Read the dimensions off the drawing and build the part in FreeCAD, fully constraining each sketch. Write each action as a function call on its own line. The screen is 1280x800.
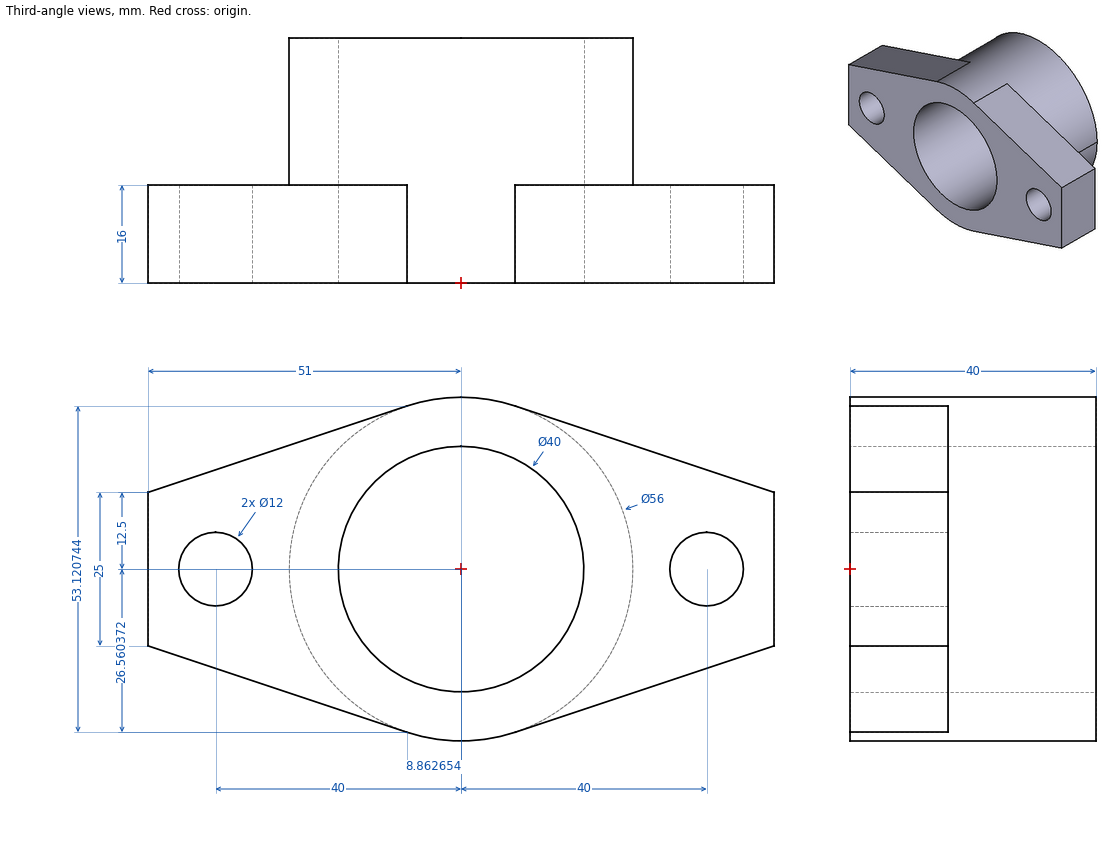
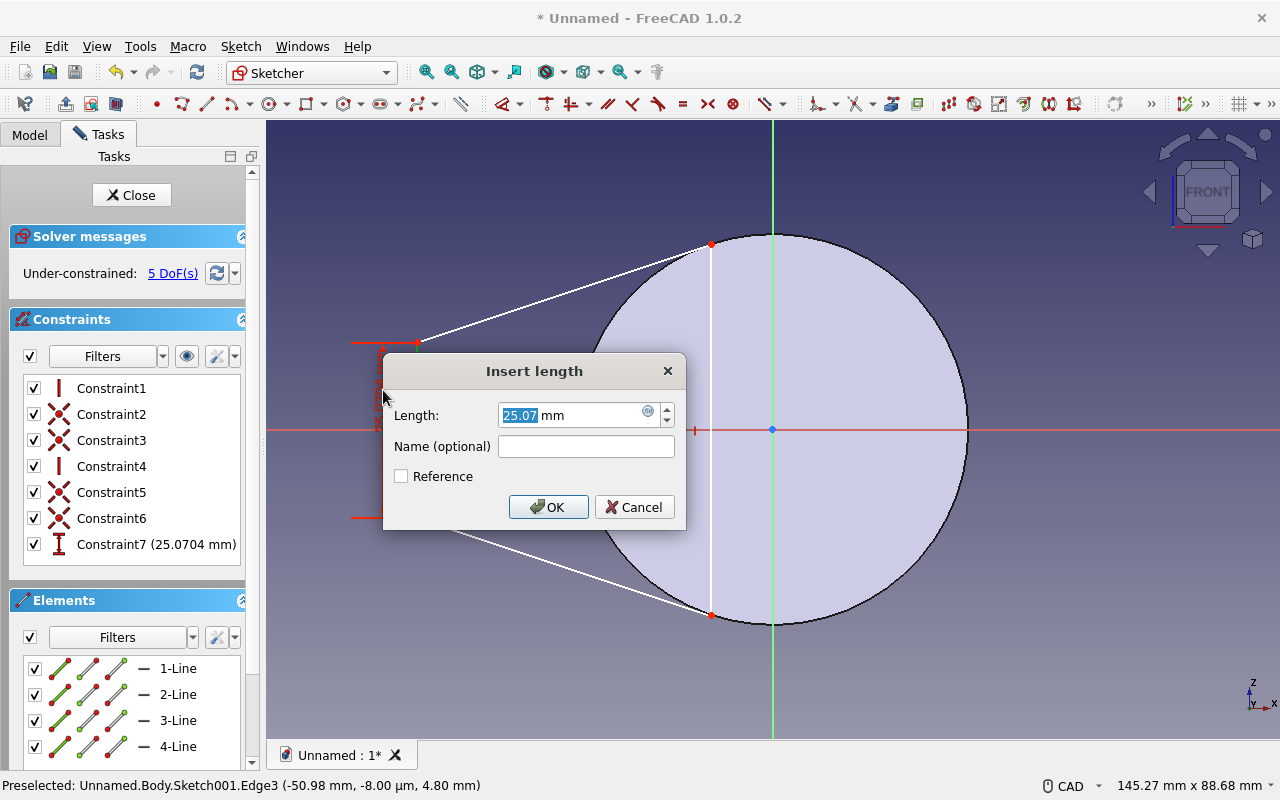
text(25)
key(Return)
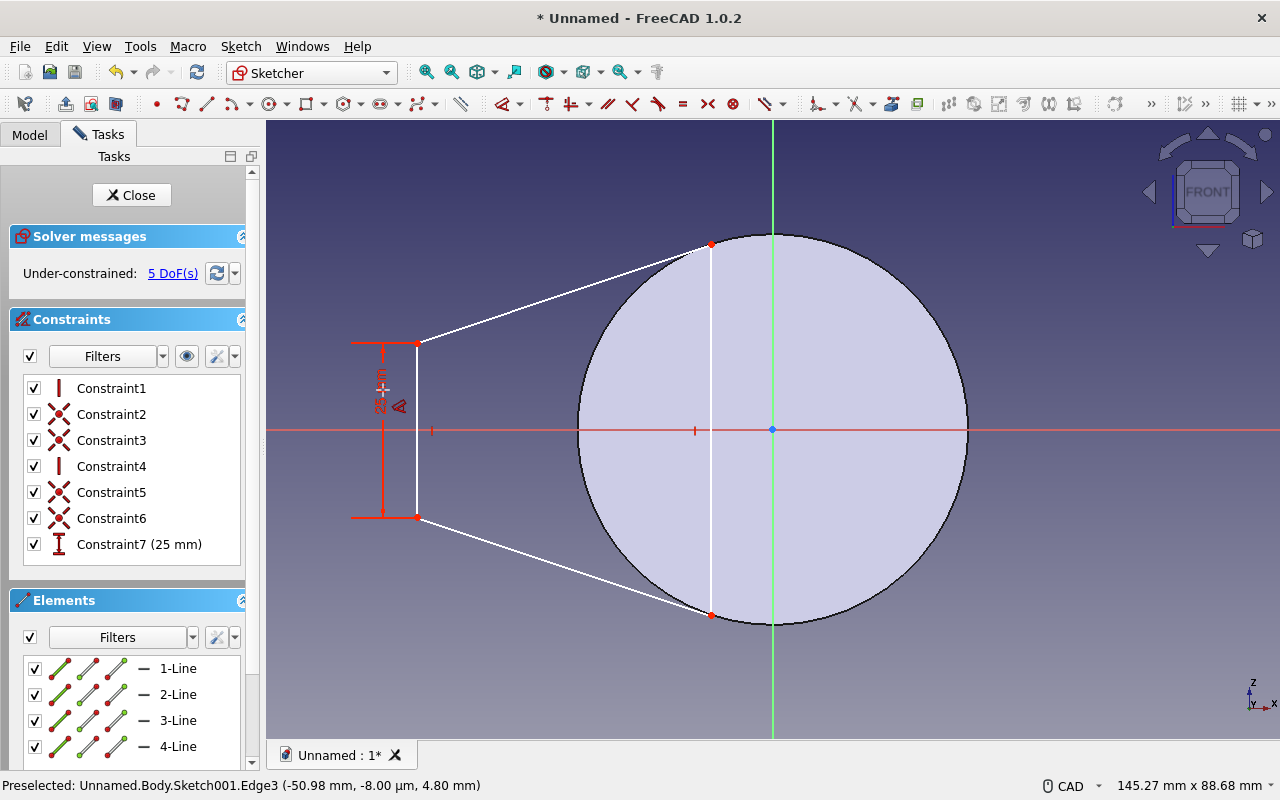
click(417, 343)
click(595, 309)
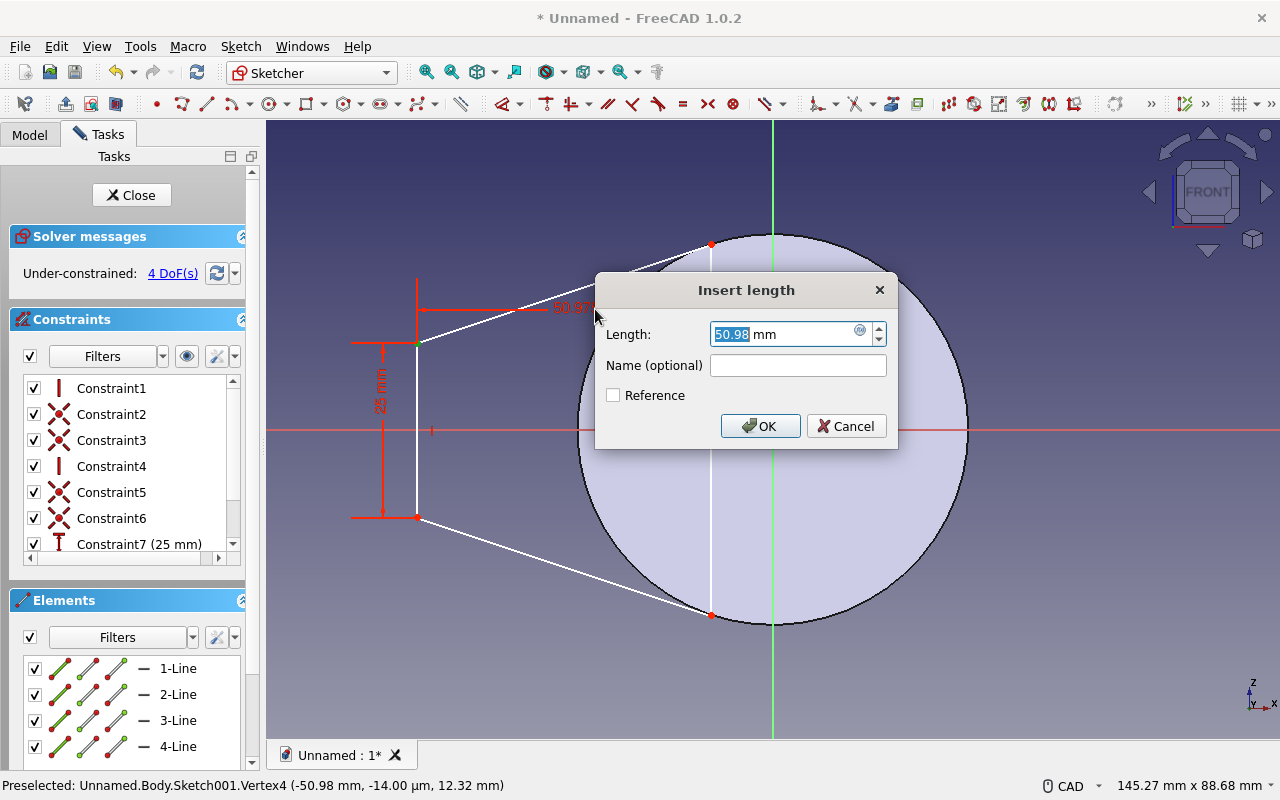
text(51)
key(Return)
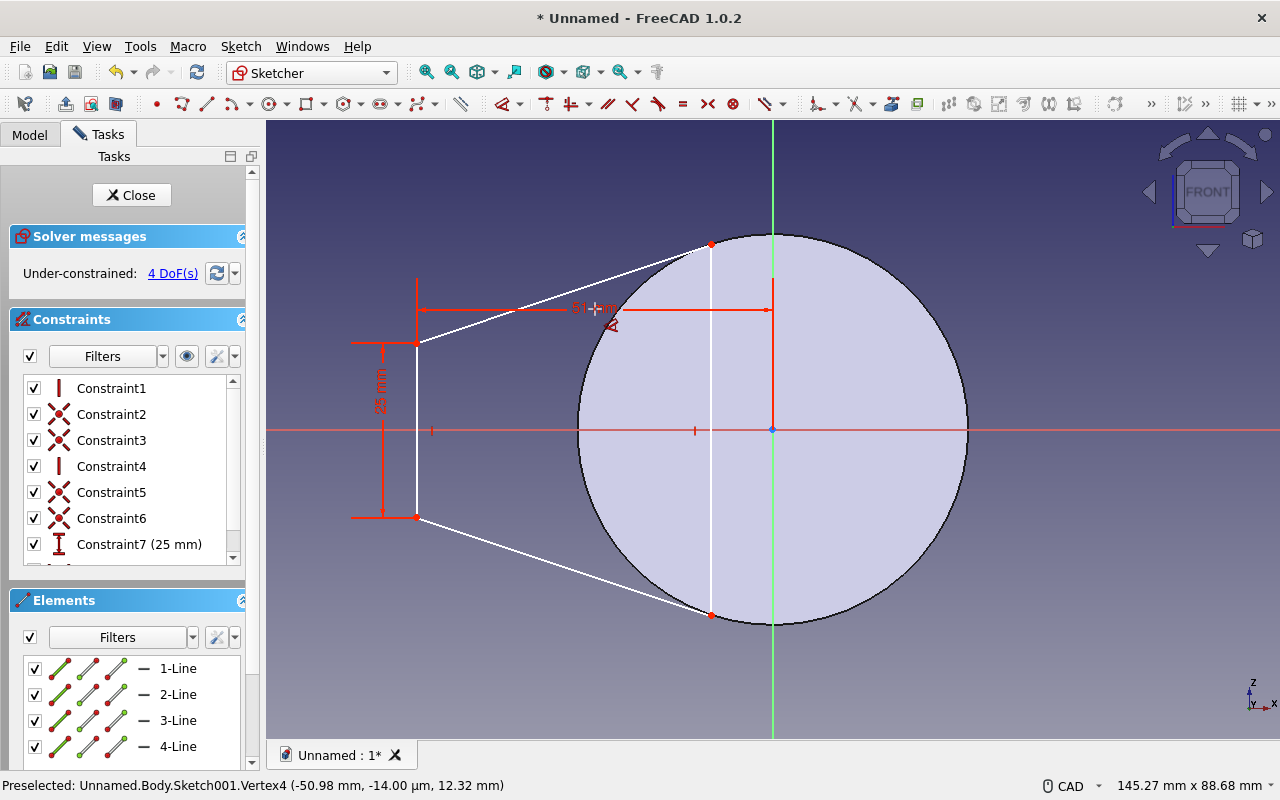
click(417, 343)
click(807, 386)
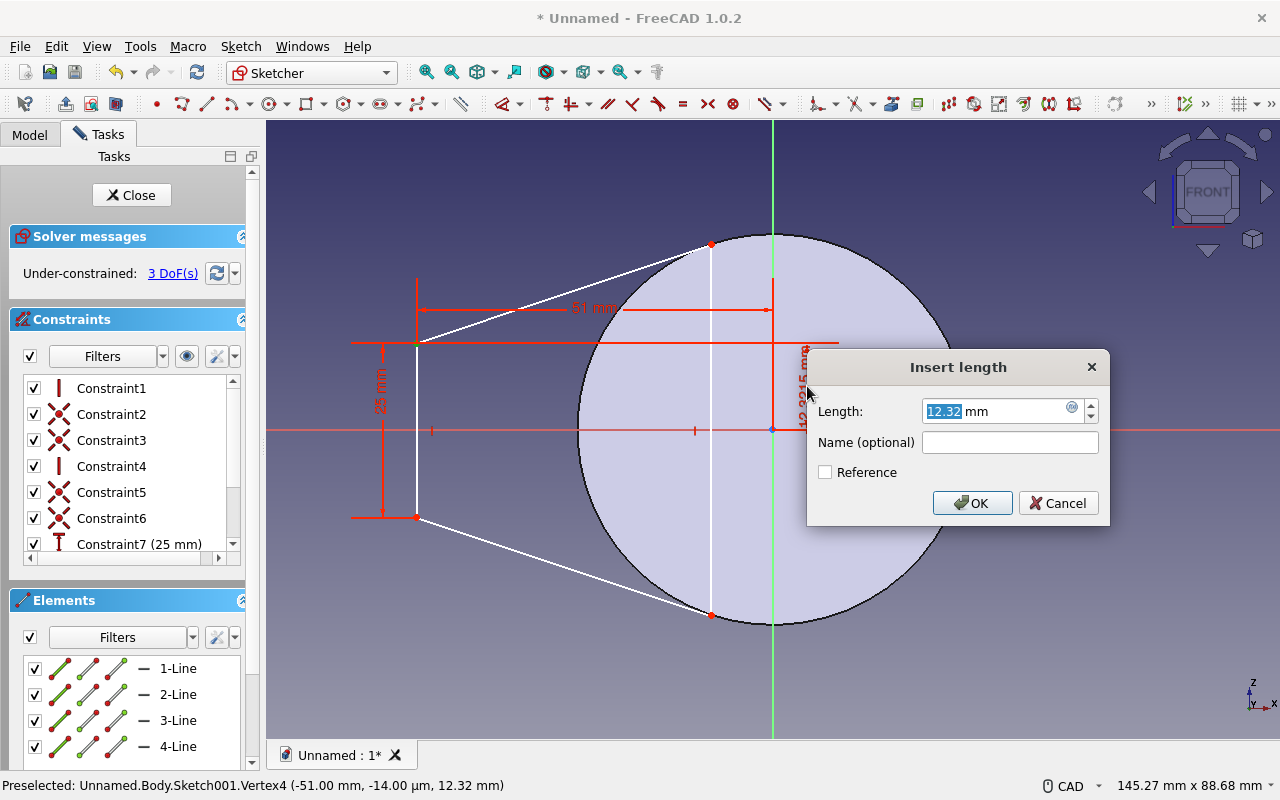
text(12.5)
key(Return)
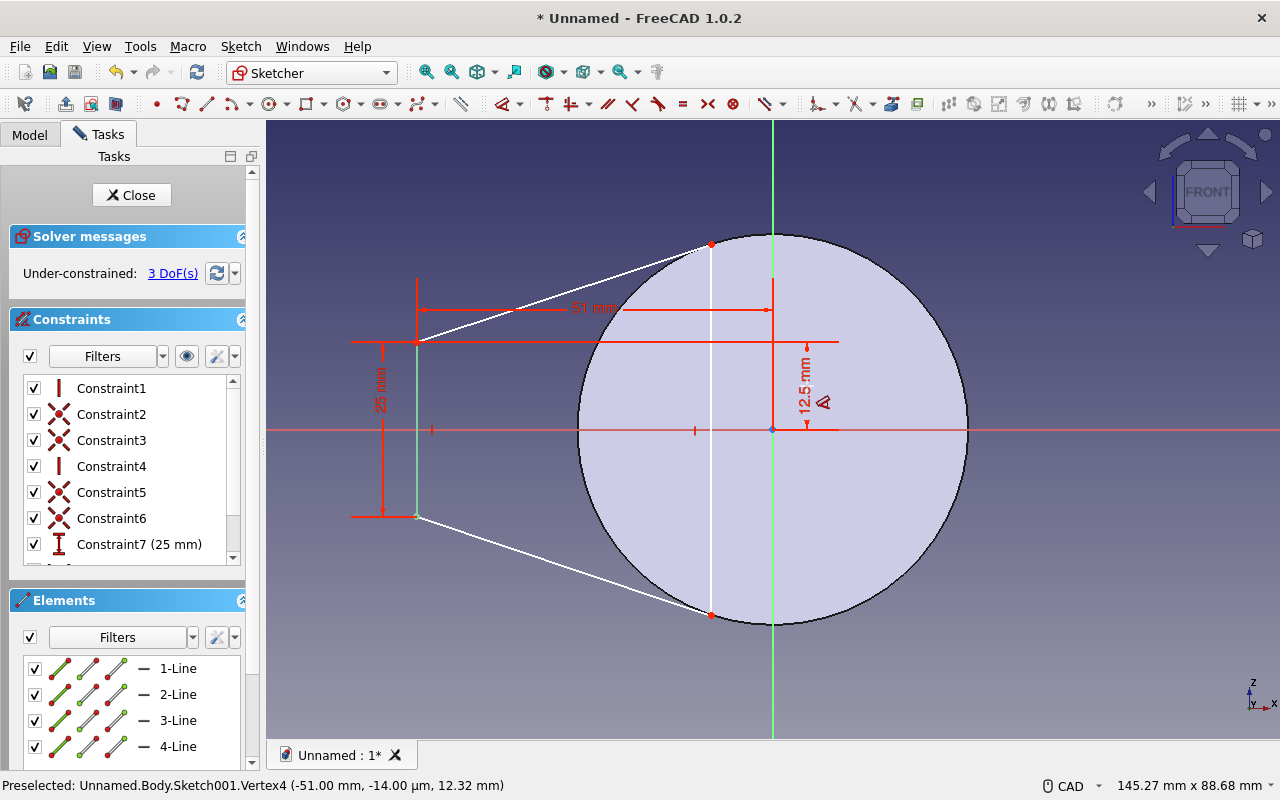
click(711, 505)
click(745, 345)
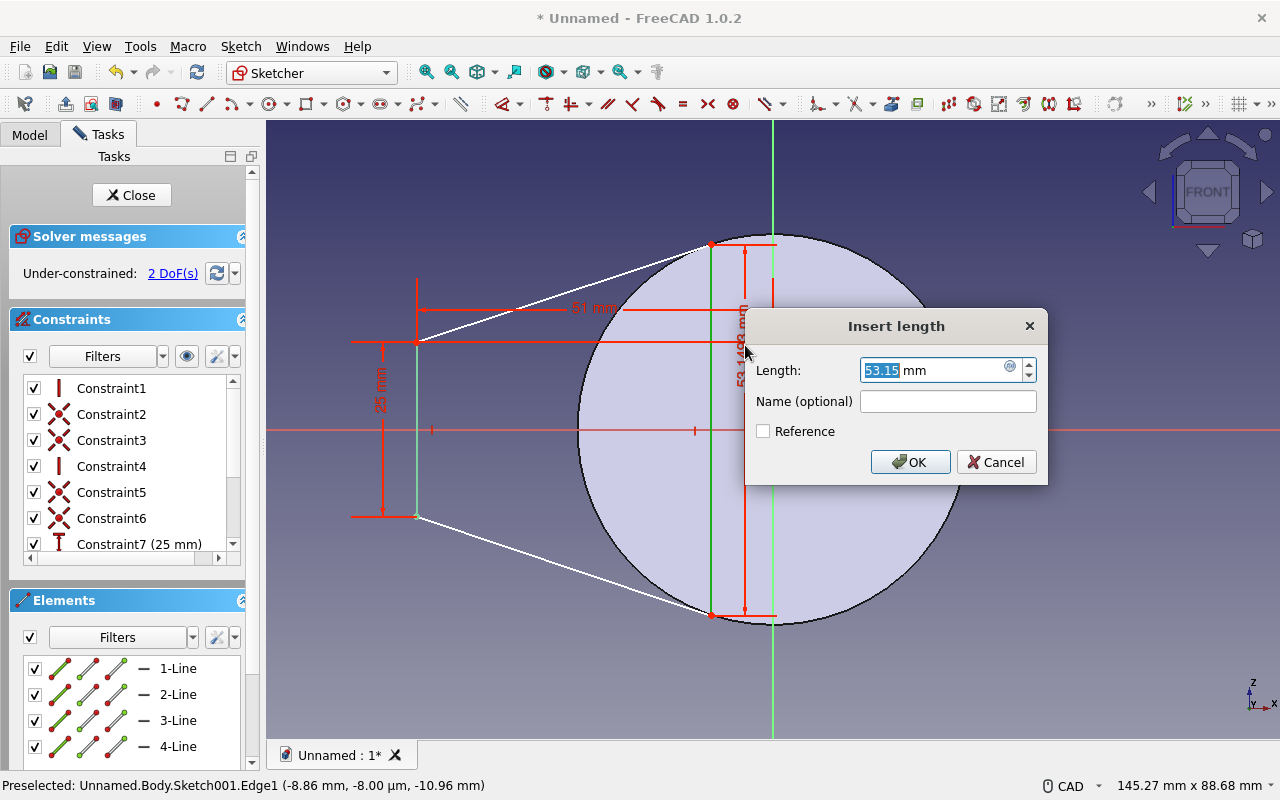
text(53.120744)
key(Return)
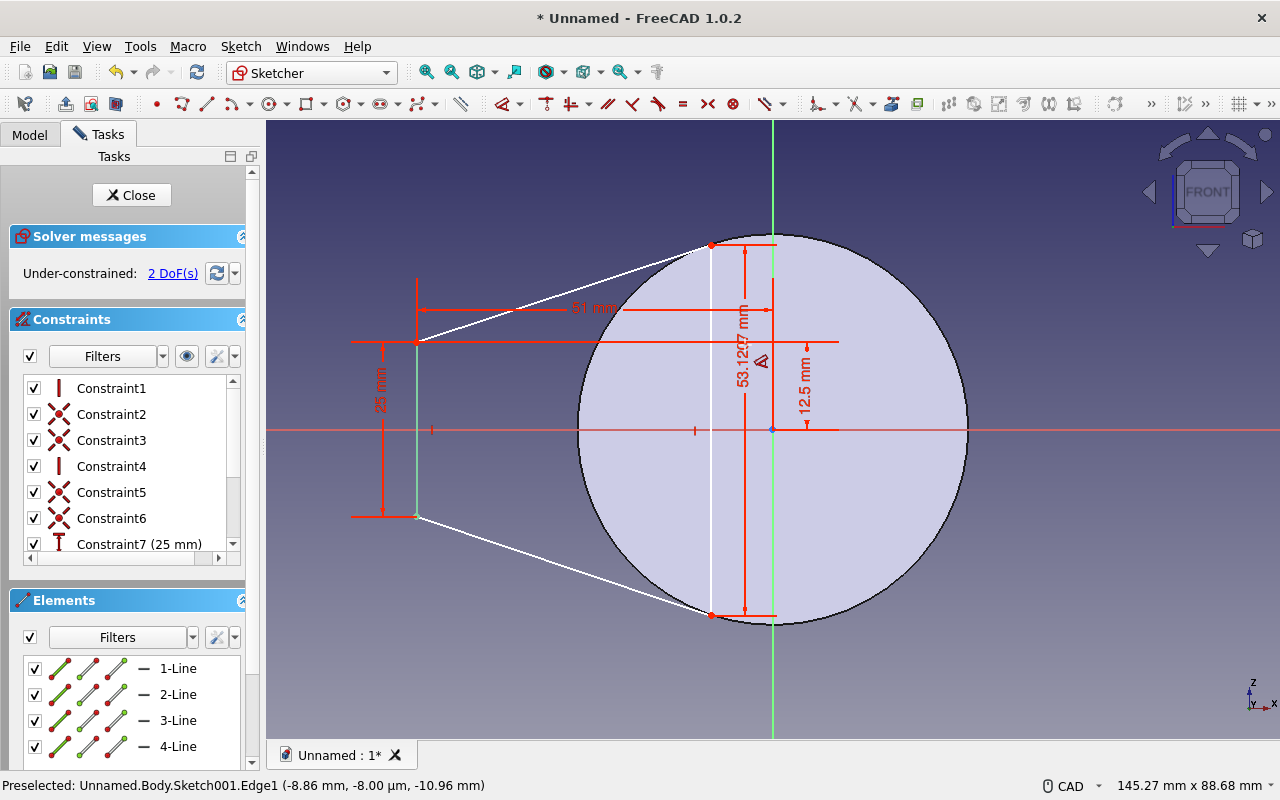
click(711, 616)
click(742, 650)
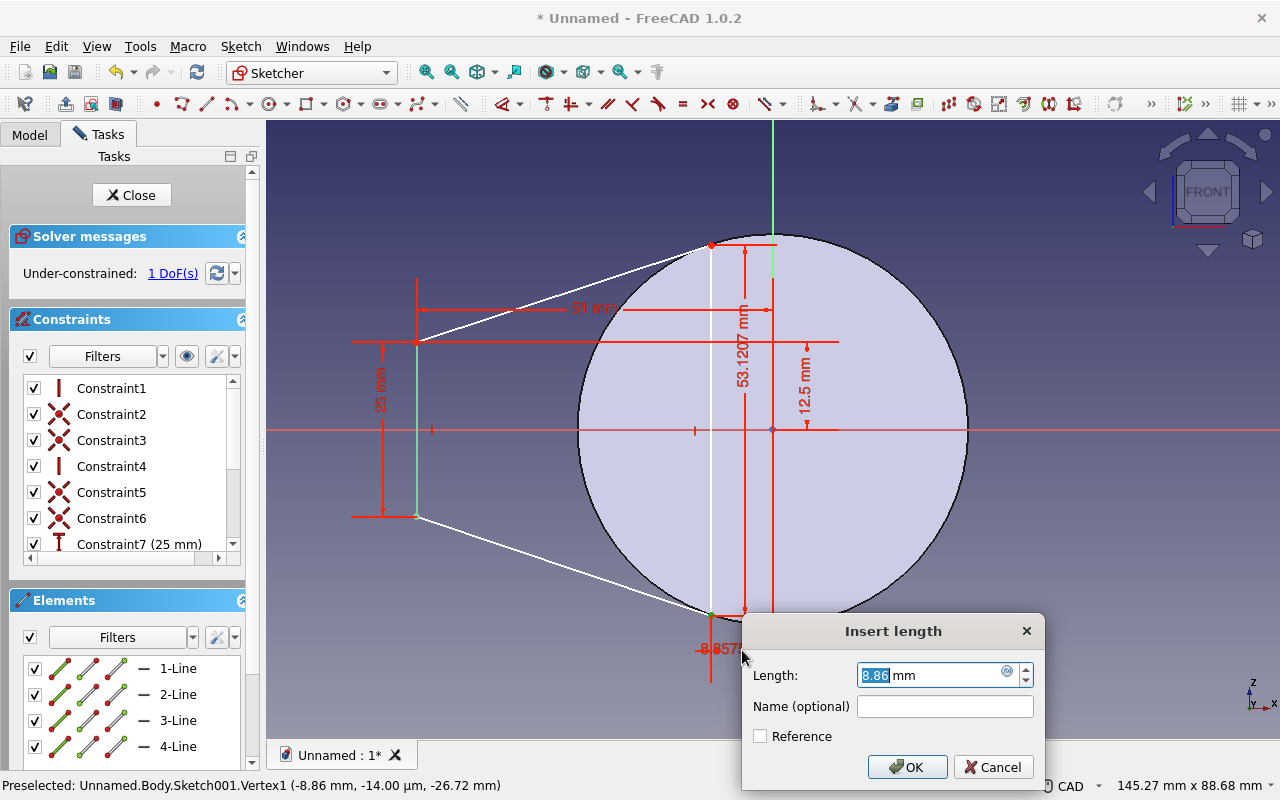
text(8.862654)
key(Return)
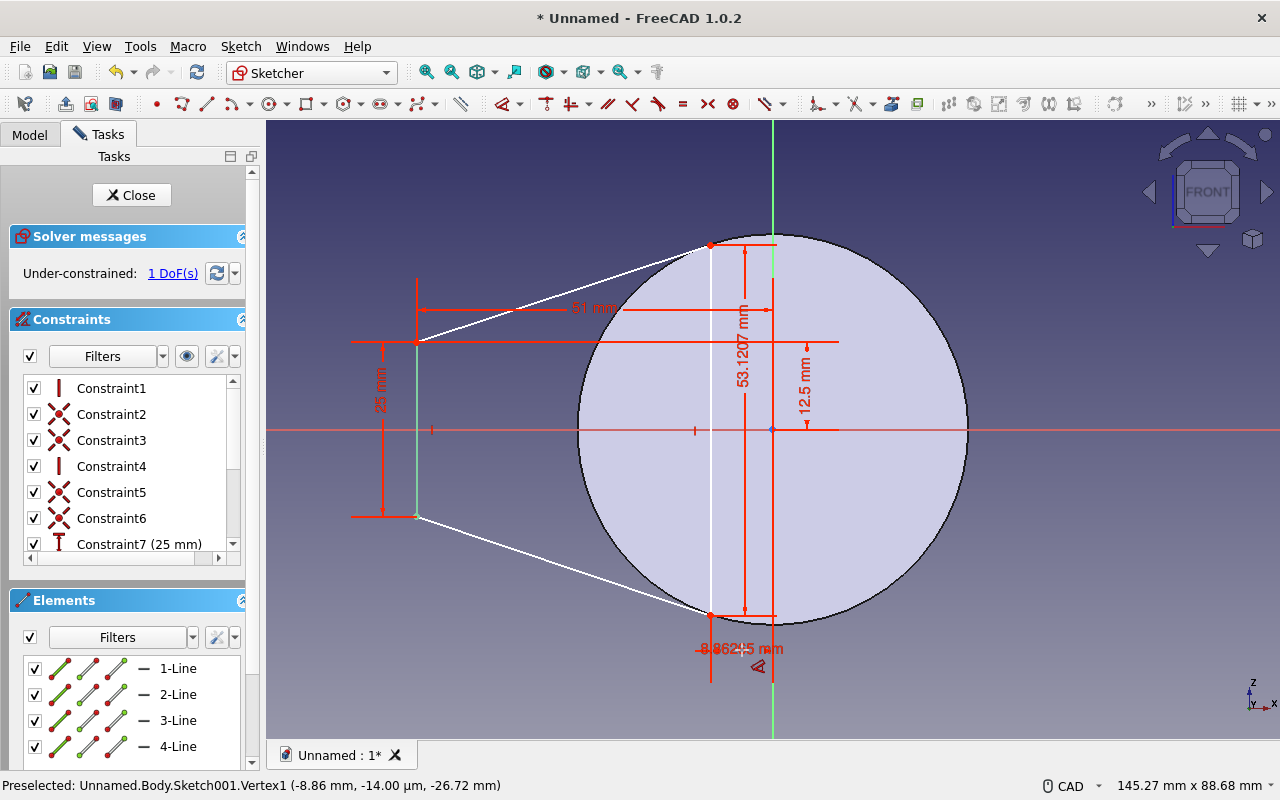
click(711, 616)
click(807, 523)